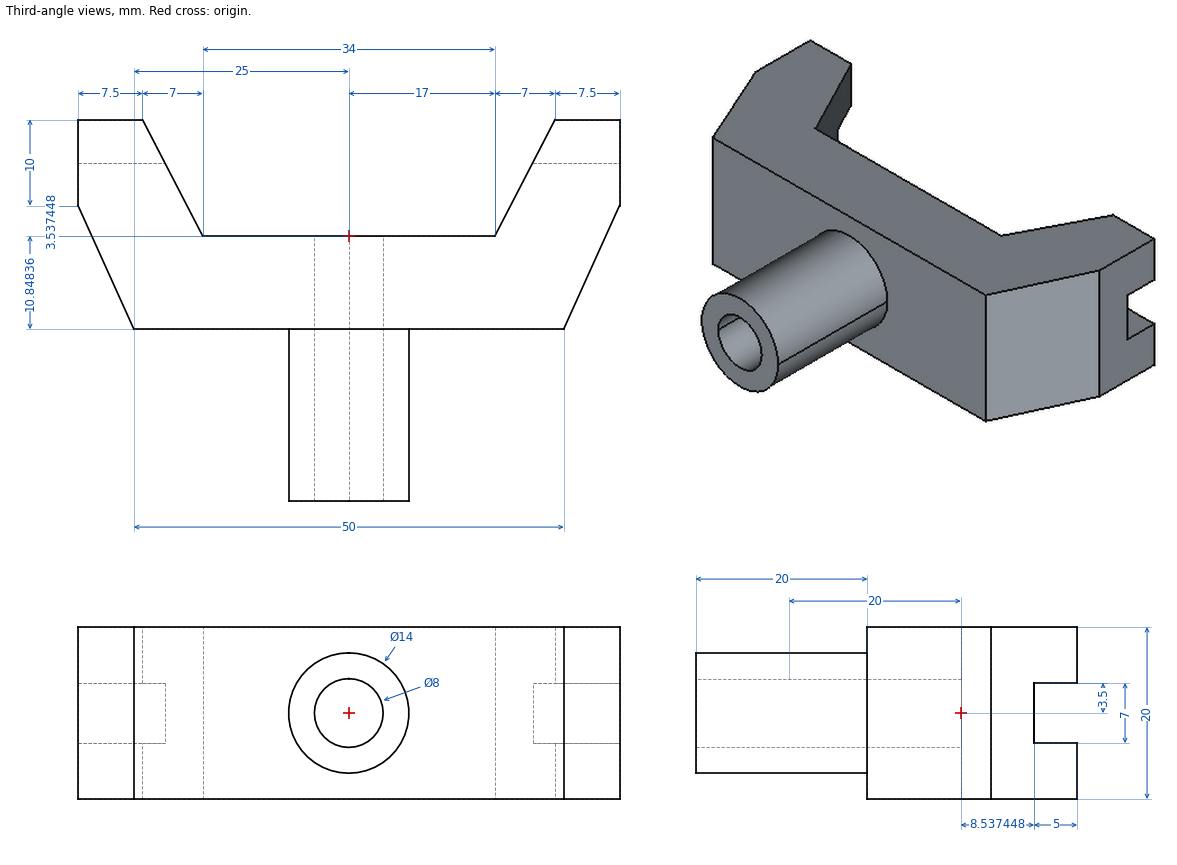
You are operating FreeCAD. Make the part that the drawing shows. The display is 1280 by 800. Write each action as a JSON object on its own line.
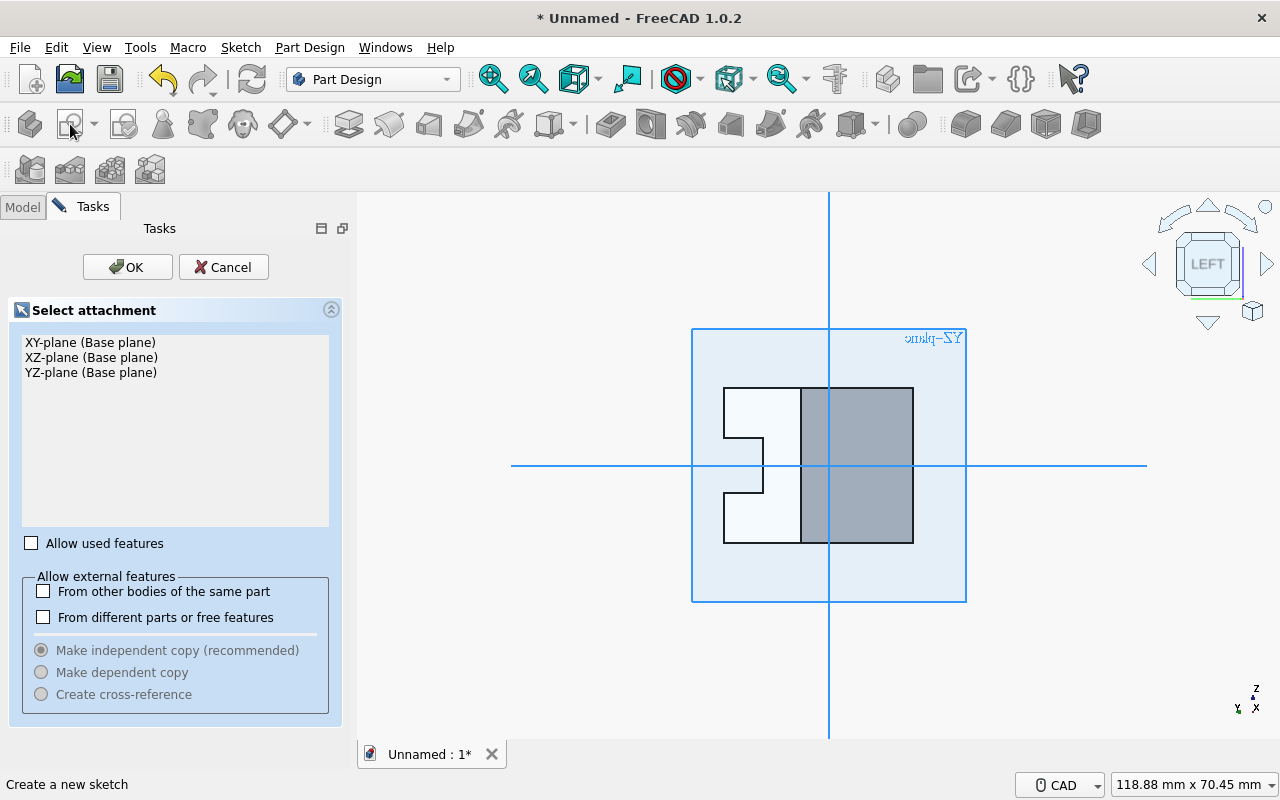
{"action": "left_click", "coordinate": [82, 358]}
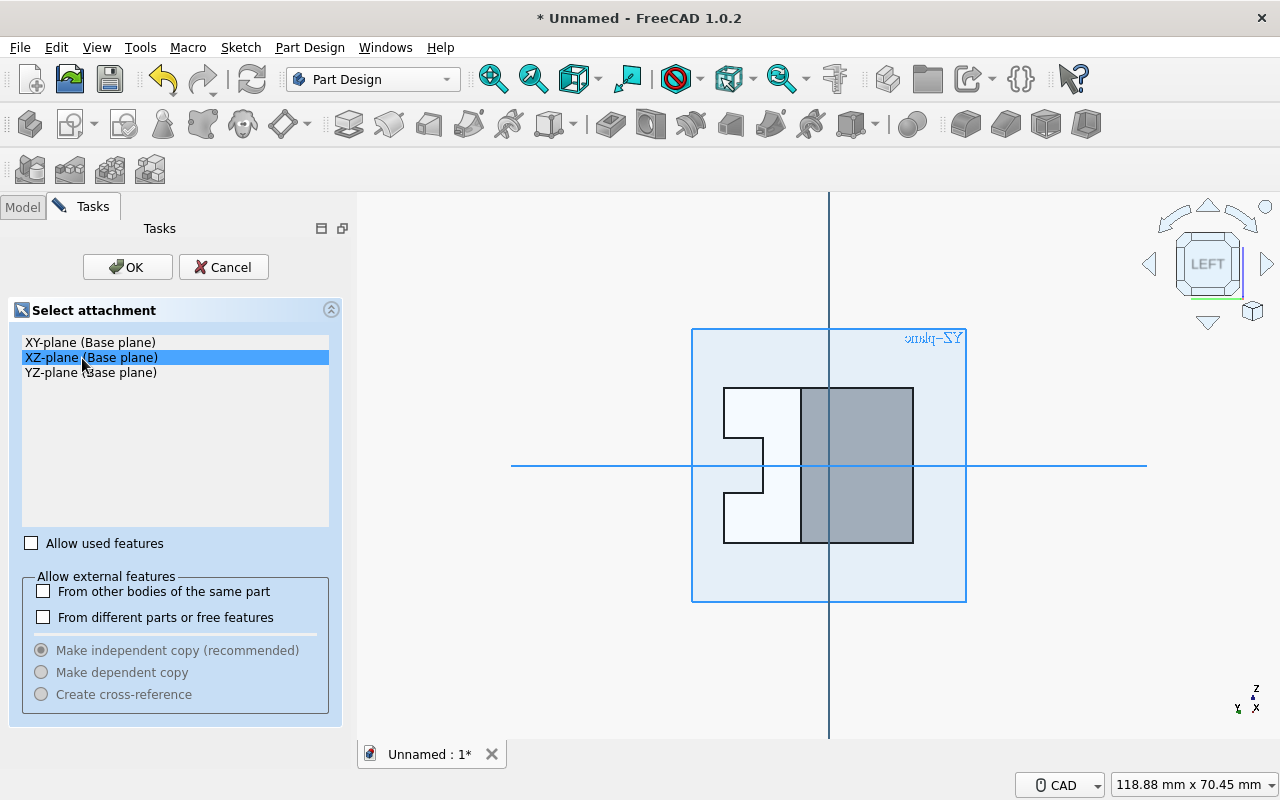
{"action": "left_click", "coordinate": [128, 267]}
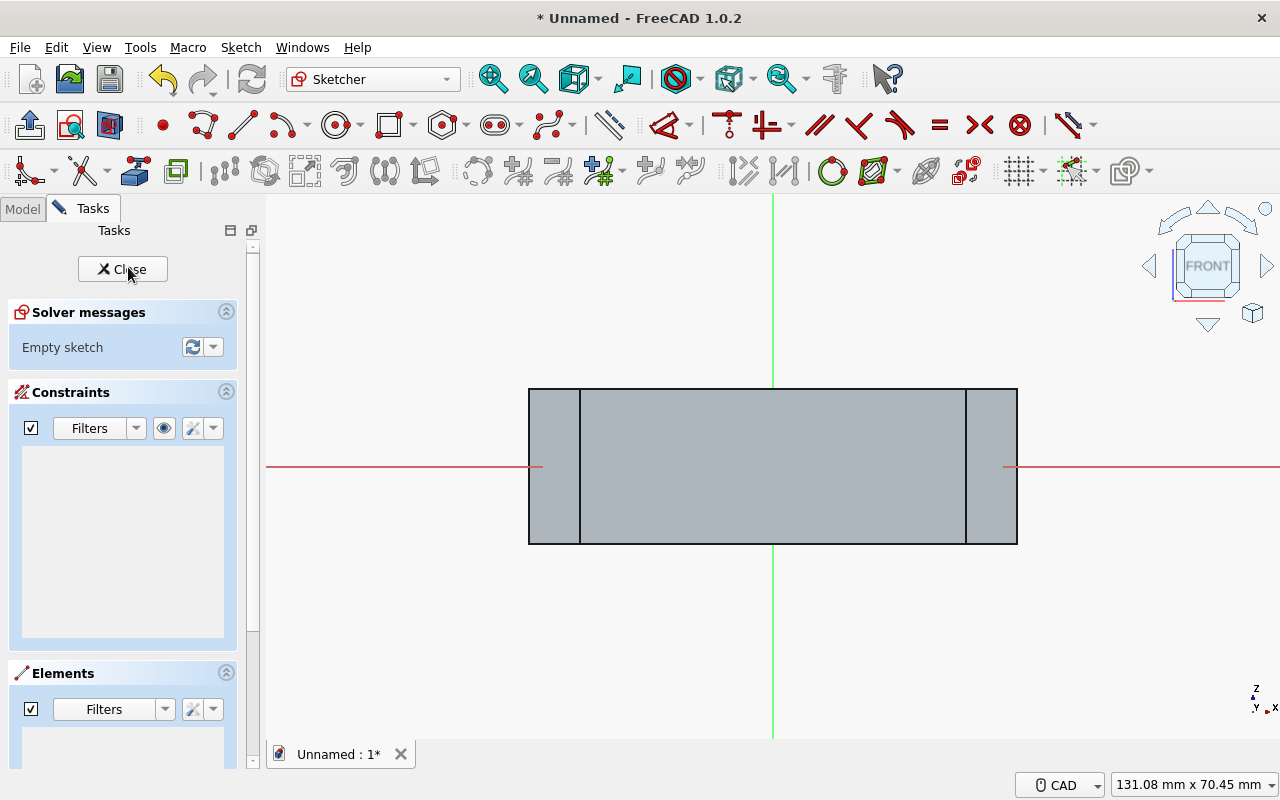
{"action": "left_click", "coordinate": [110, 126]}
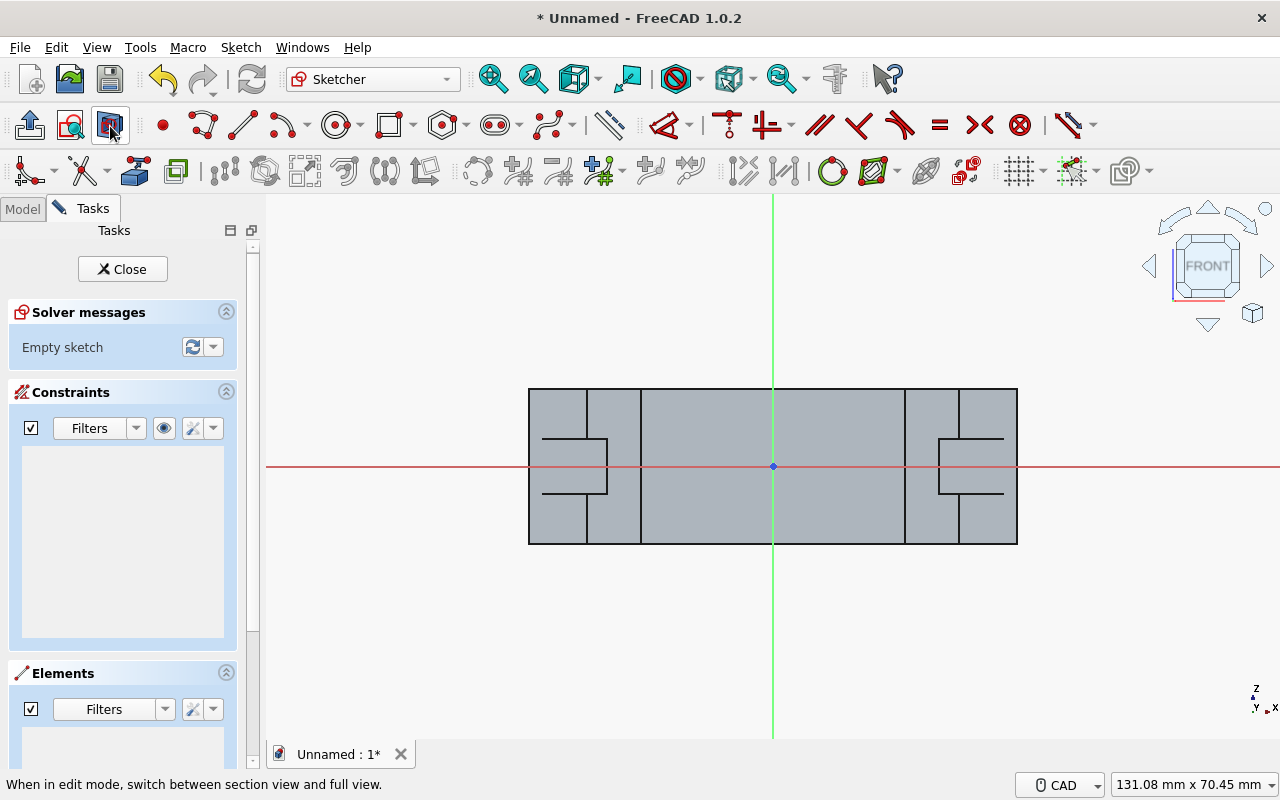
{"action": "scroll", "coordinate": [787, 467], "scroll_direction": "up", "scroll_amount": 9}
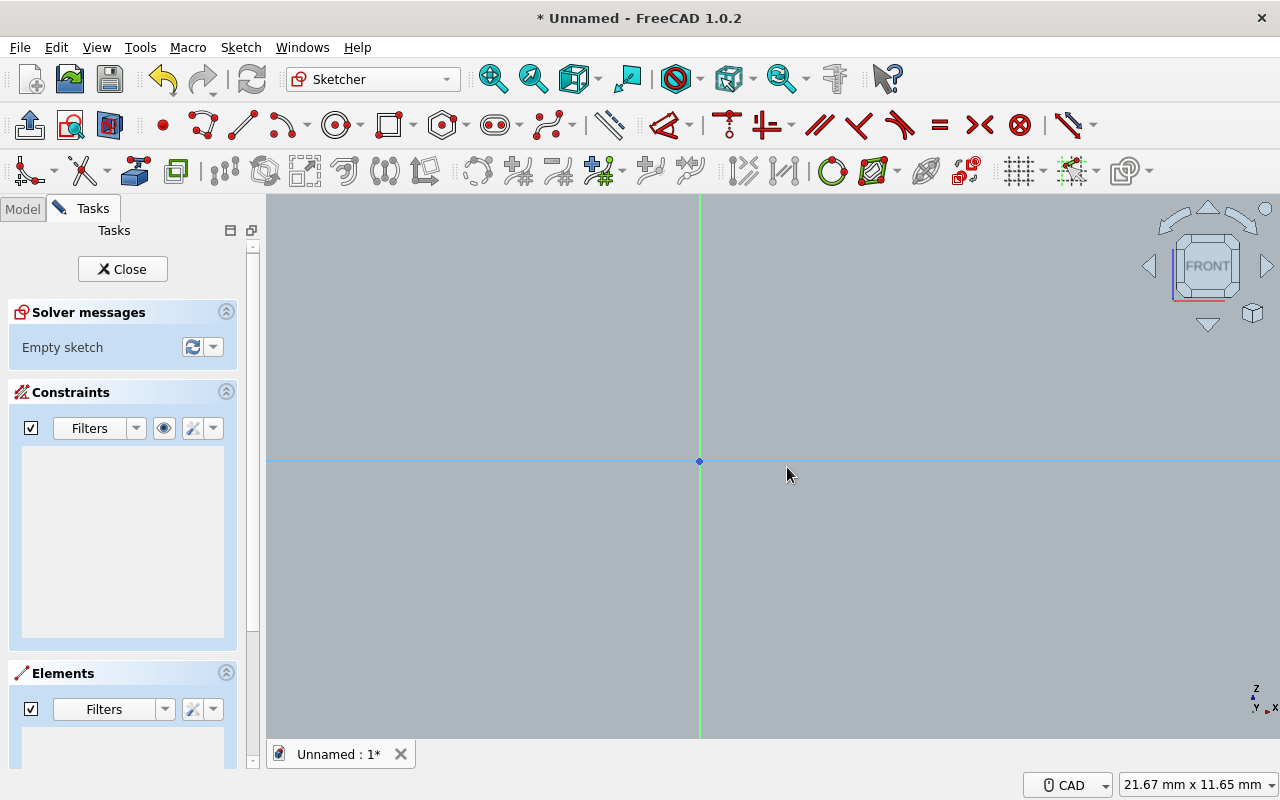
{"action": "left_click", "coordinate": [336, 126]}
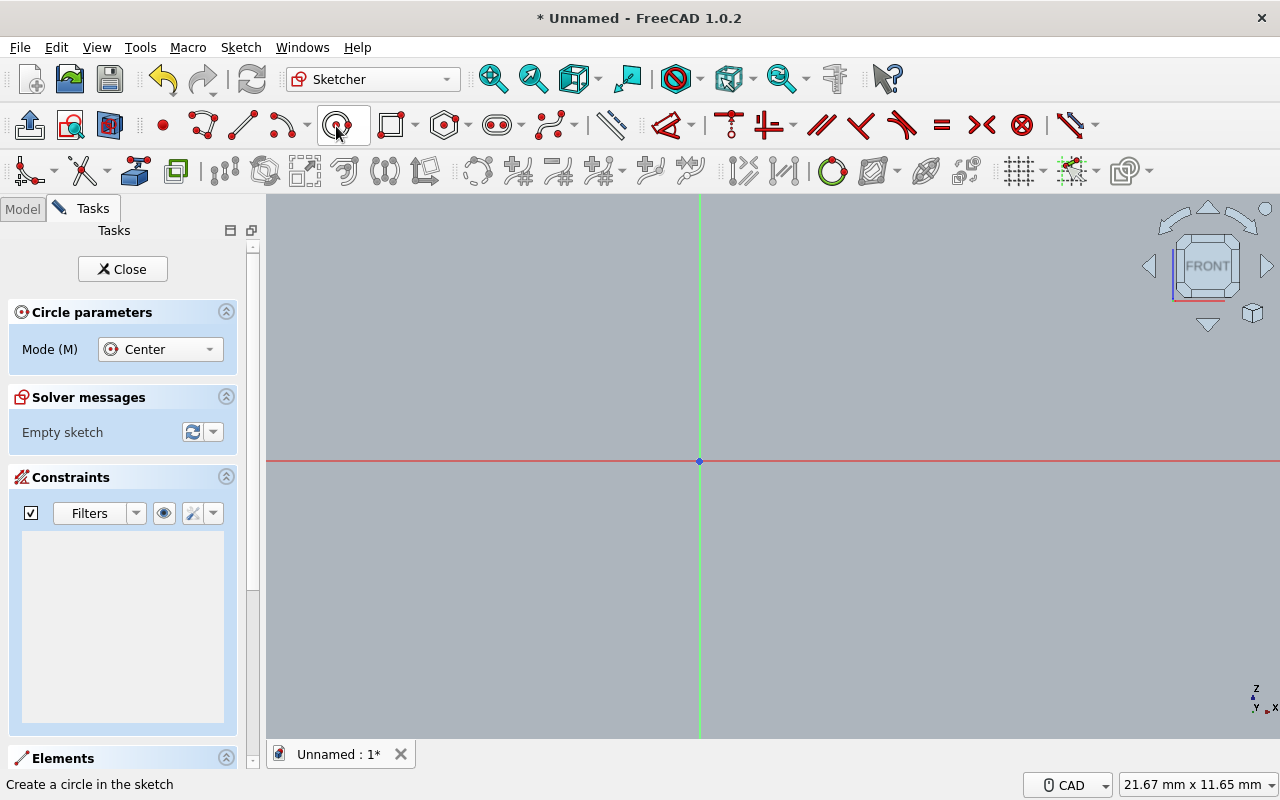
{"action": "left_click", "coordinate": [700, 461]}
{"action": "mouse_move", "coordinate": [832, 329]}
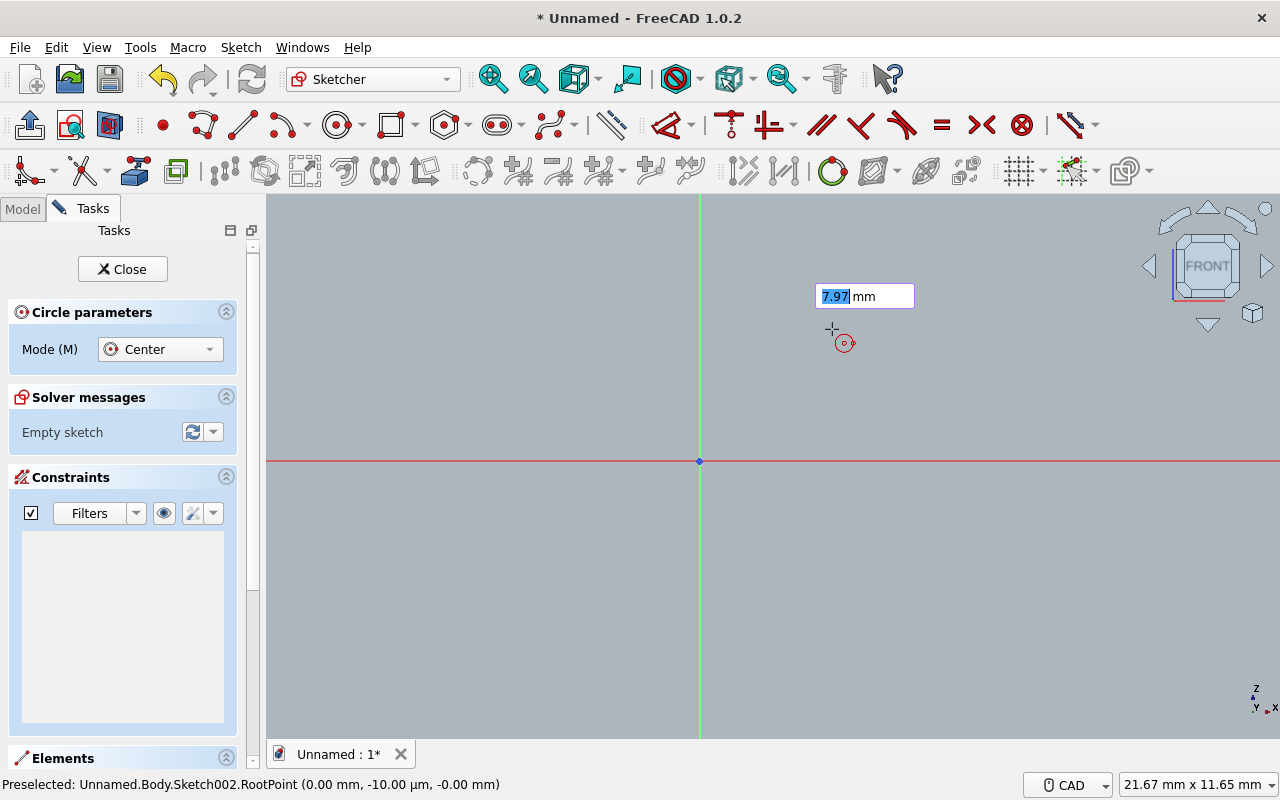
{"action": "type", "text": "8"}
{"action": "key", "text": "Return"}
{"action": "key", "text": "Escape"}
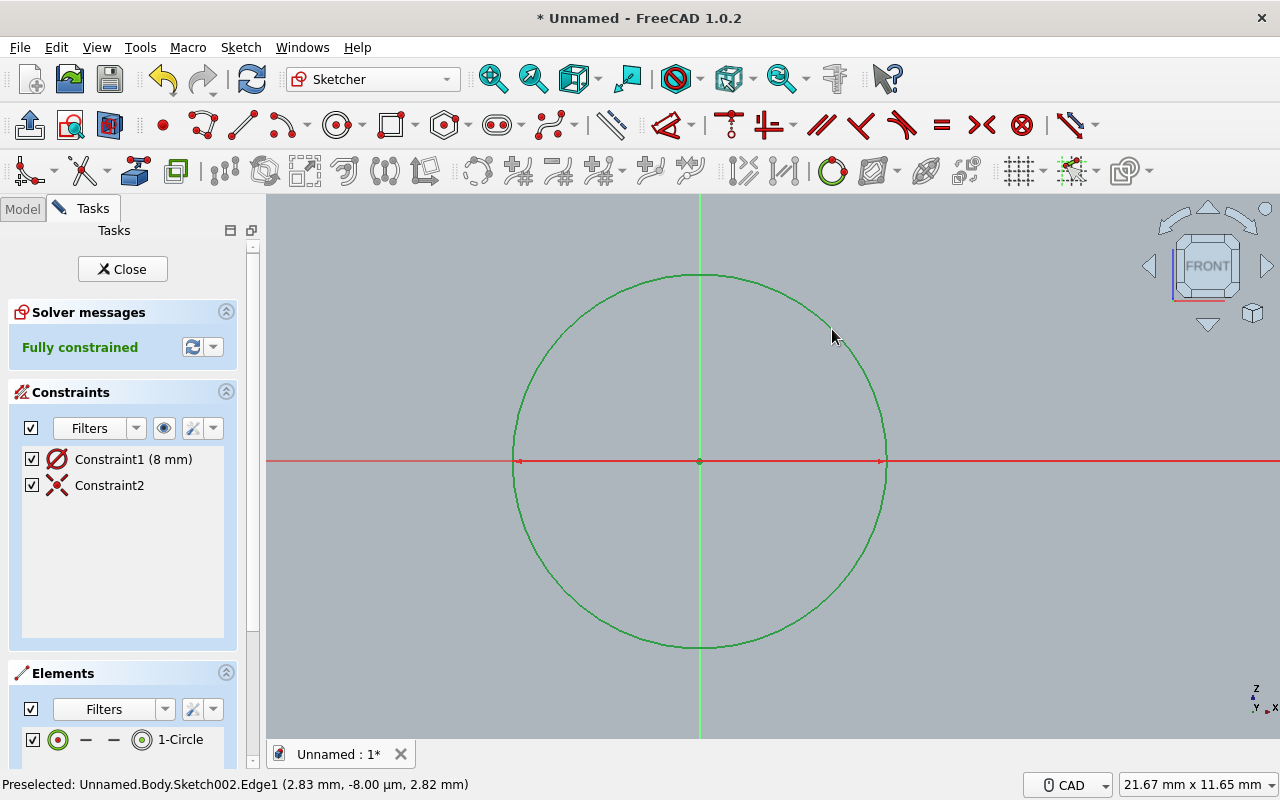
{"action": "left_click", "coordinate": [123, 269]}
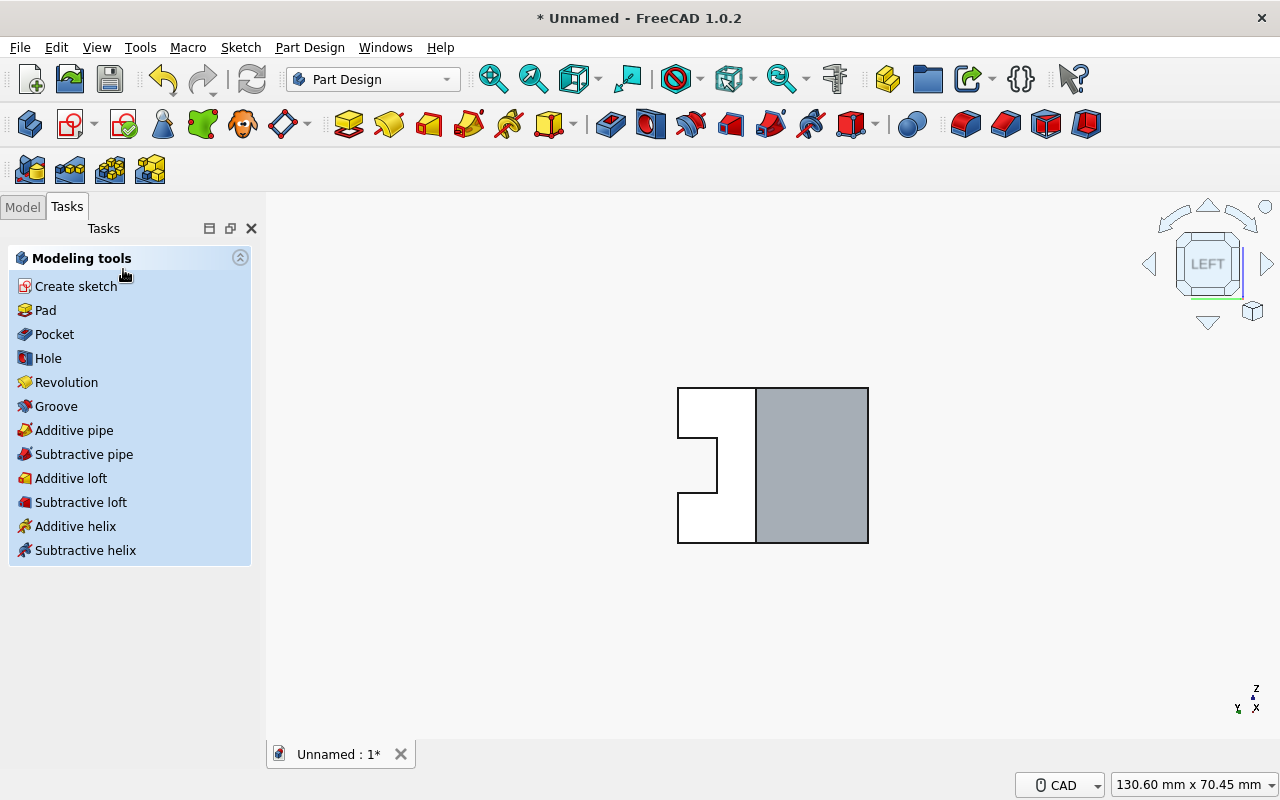
{"action": "left_click", "coordinate": [612, 124]}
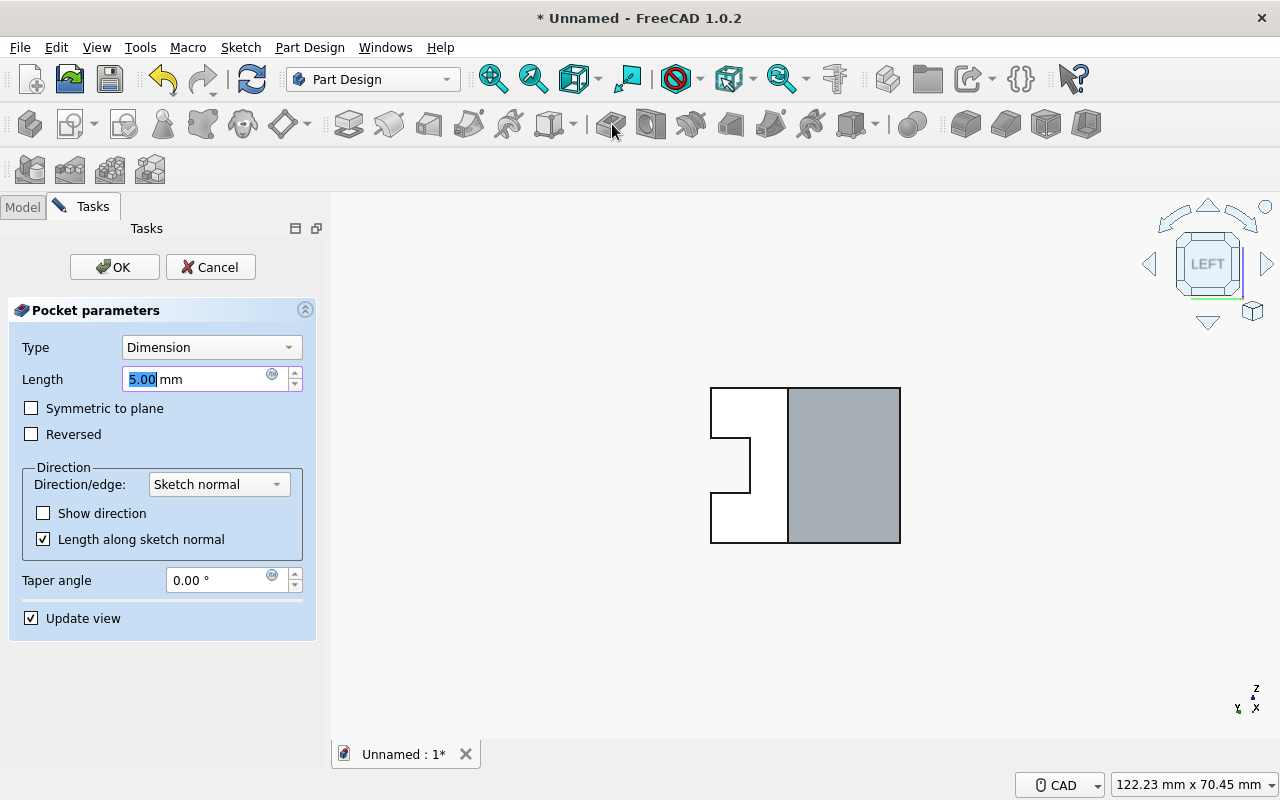
{"action": "type", "text": "20"}
{"action": "key", "text": "Tab"}